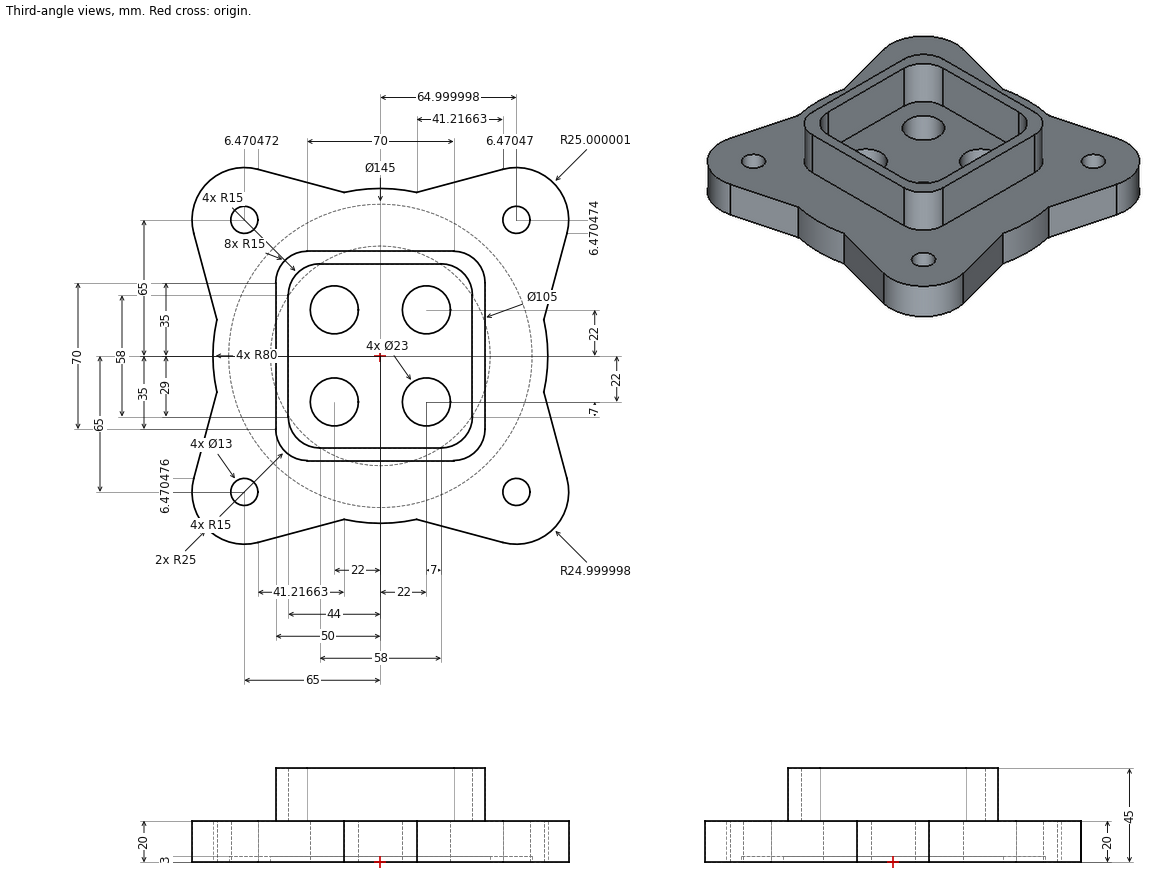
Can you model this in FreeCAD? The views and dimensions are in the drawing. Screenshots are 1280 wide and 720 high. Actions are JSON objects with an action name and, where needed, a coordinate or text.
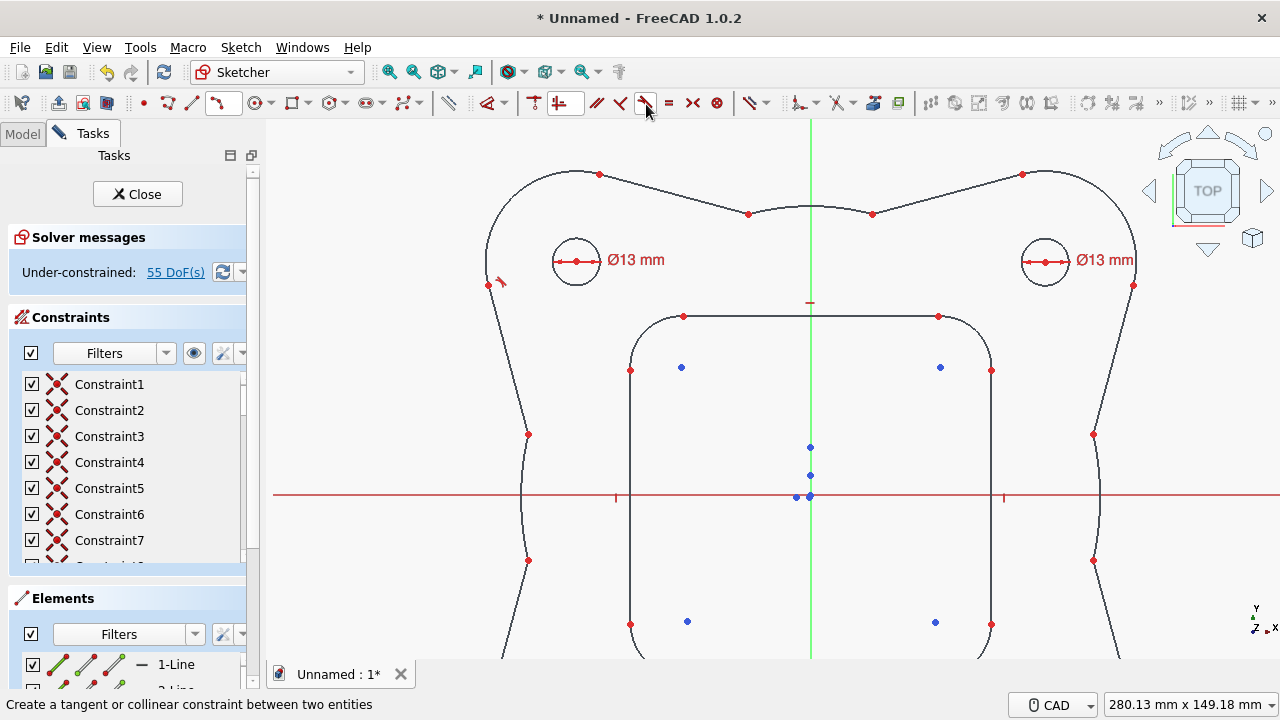
{"action": "left_click", "coordinate": [516, 605]}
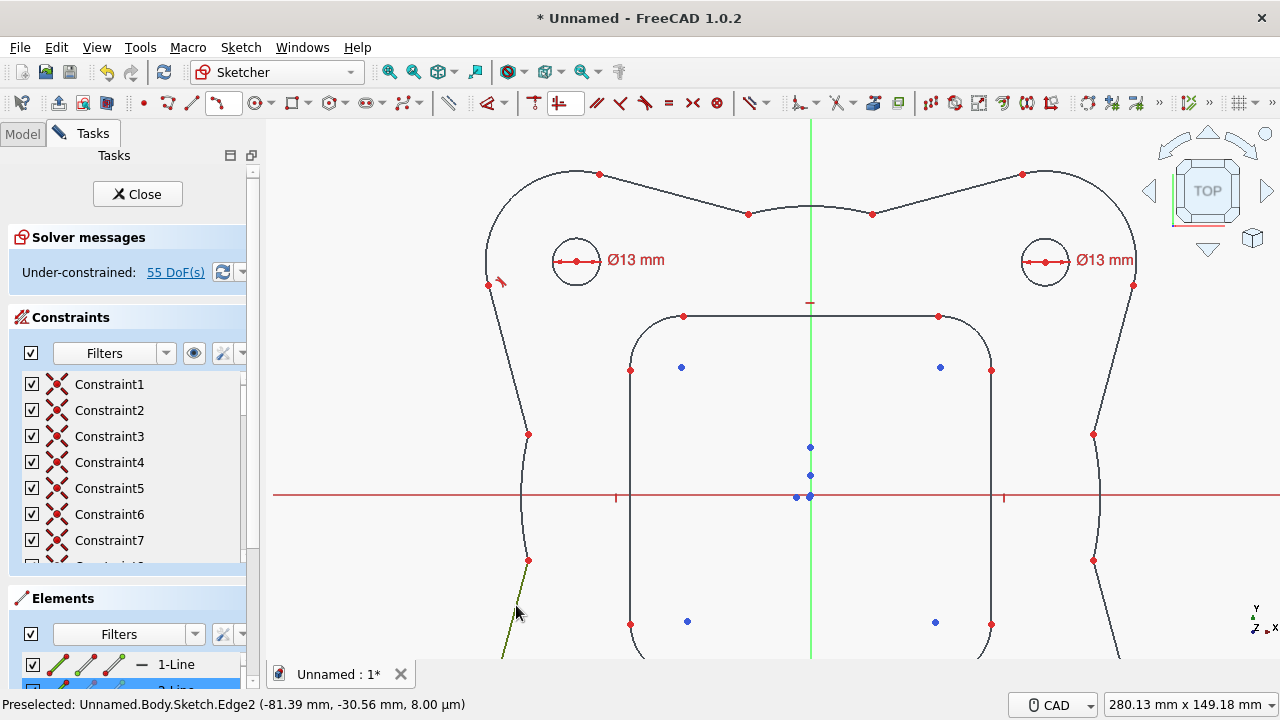
{"action": "scroll", "coordinate": [575, 260], "scroll_direction": "down", "scroll_amount": 3}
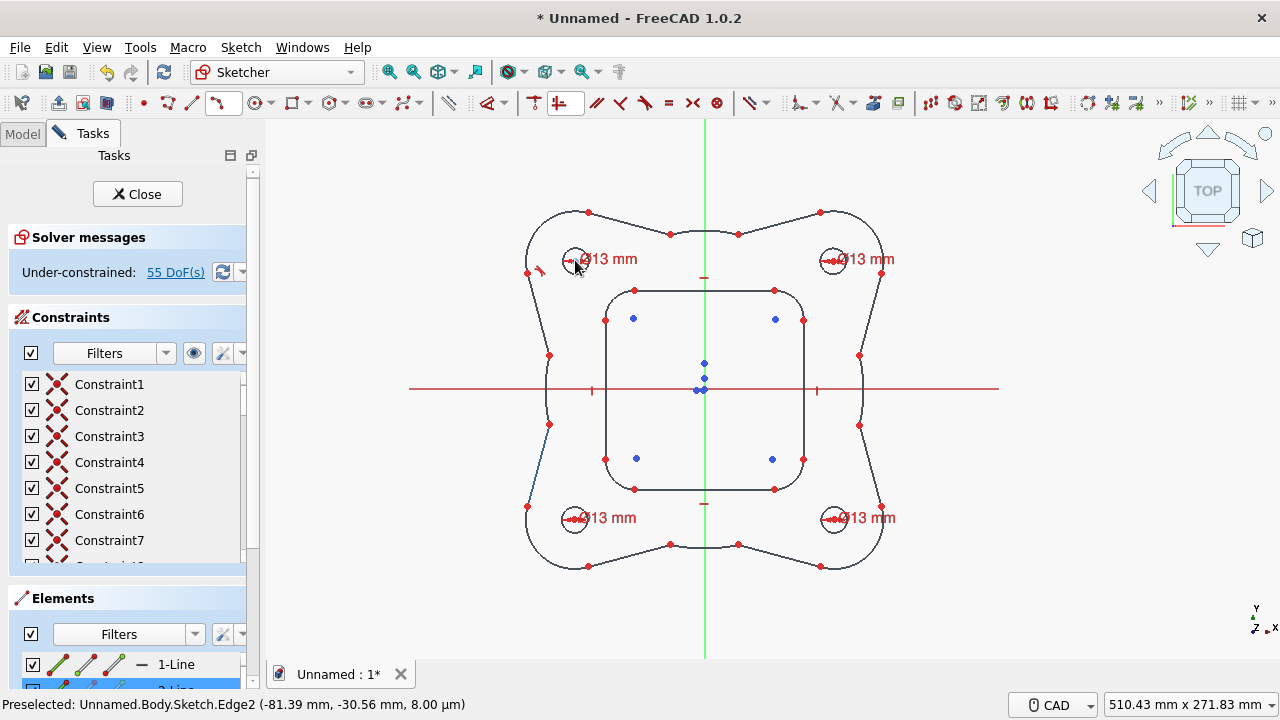
{"action": "left_click", "coordinate": [529, 538]}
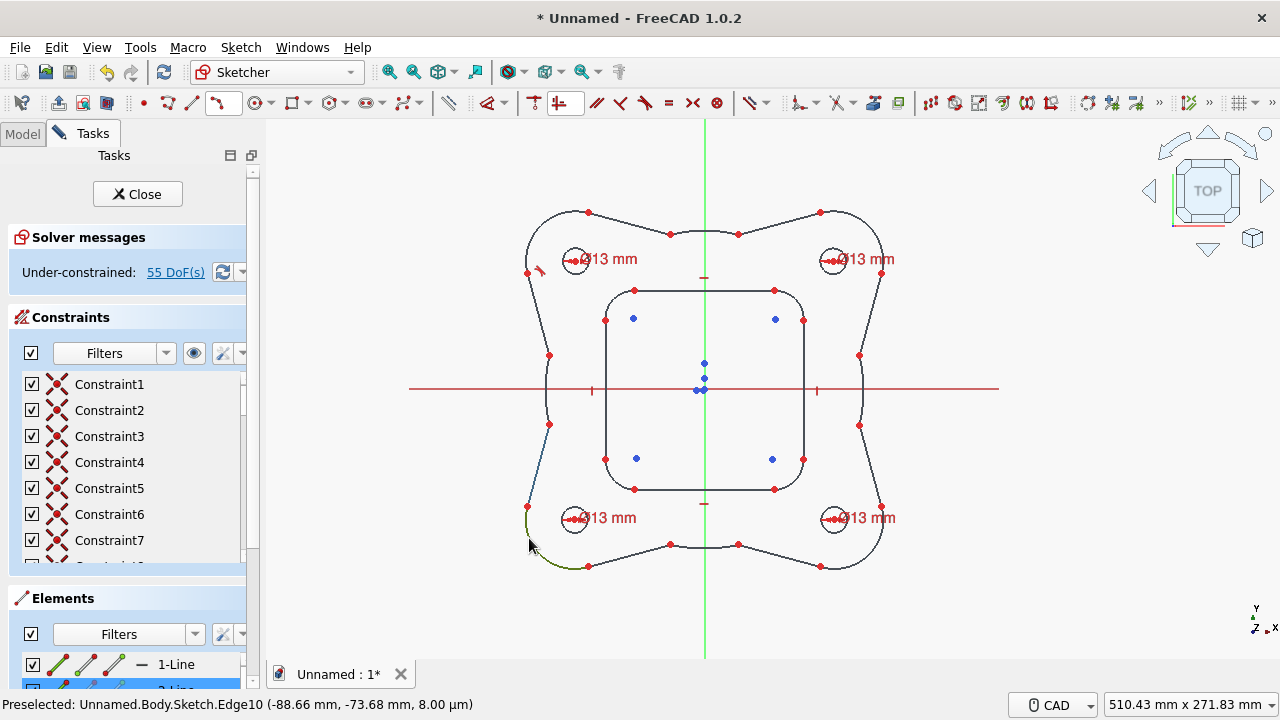
{"action": "left_click", "coordinate": [646, 104]}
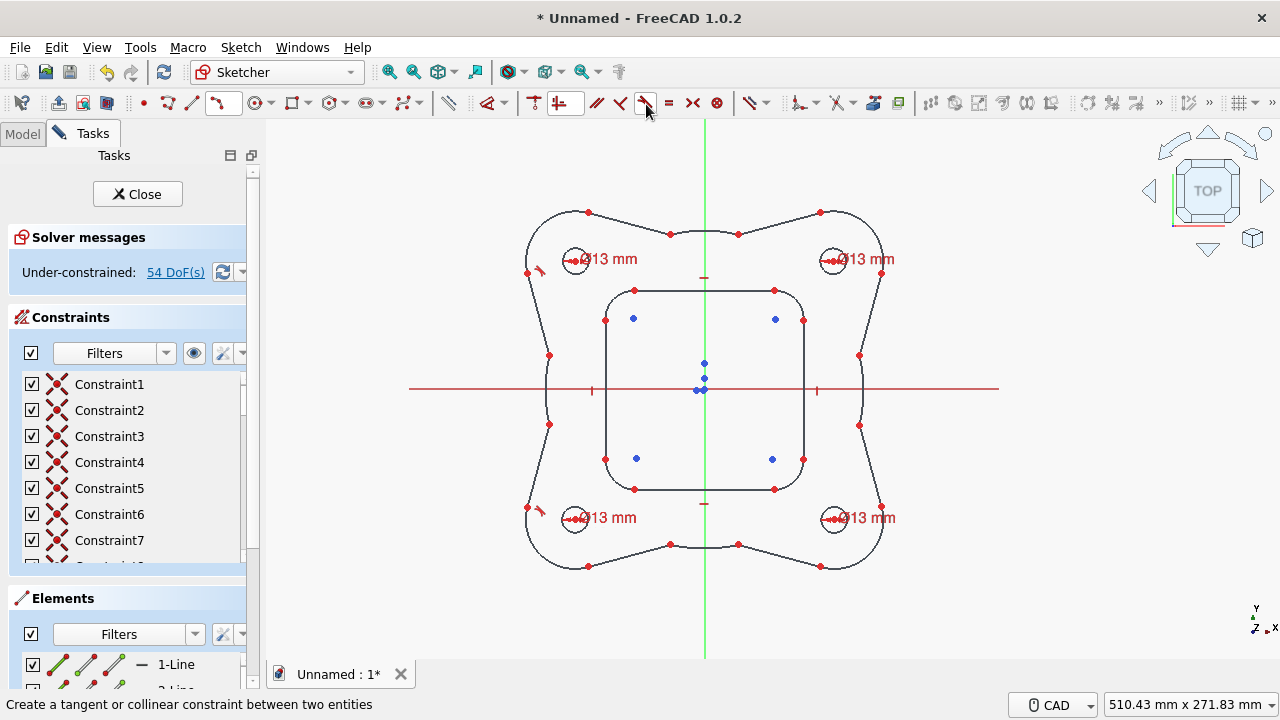
{"action": "left_click", "coordinate": [613, 560]}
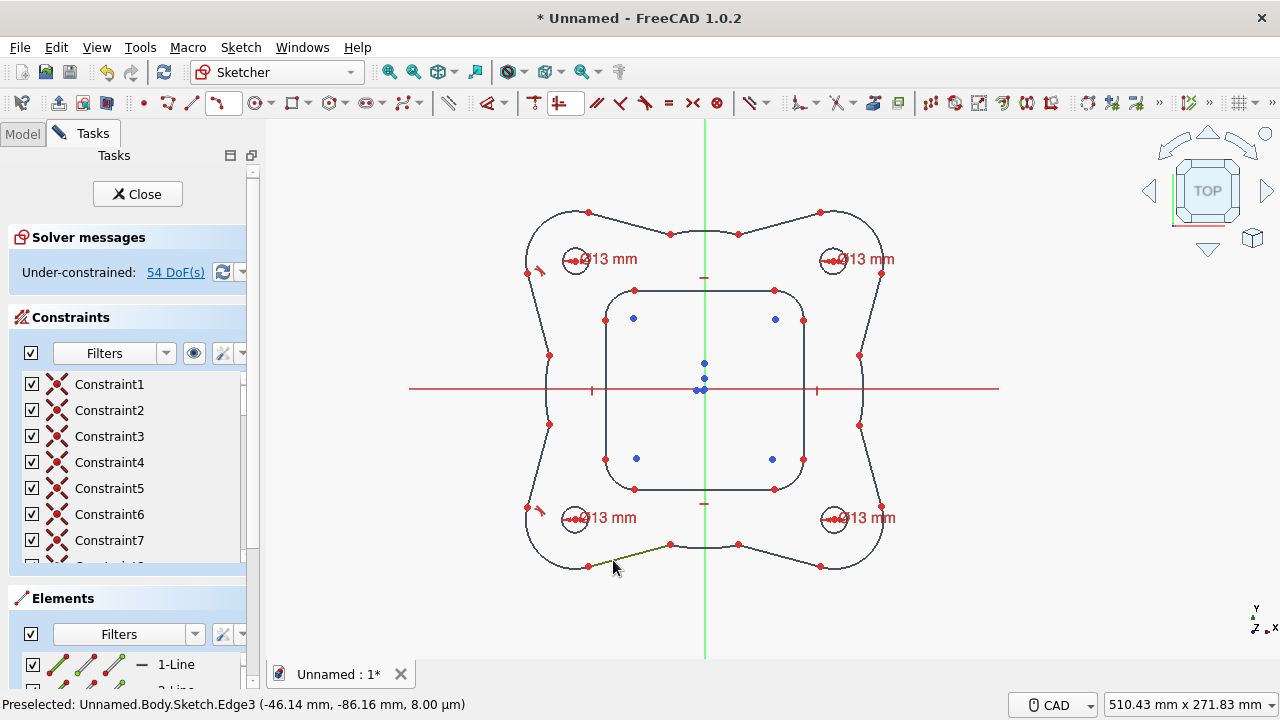
{"action": "left_click", "coordinate": [529, 538]}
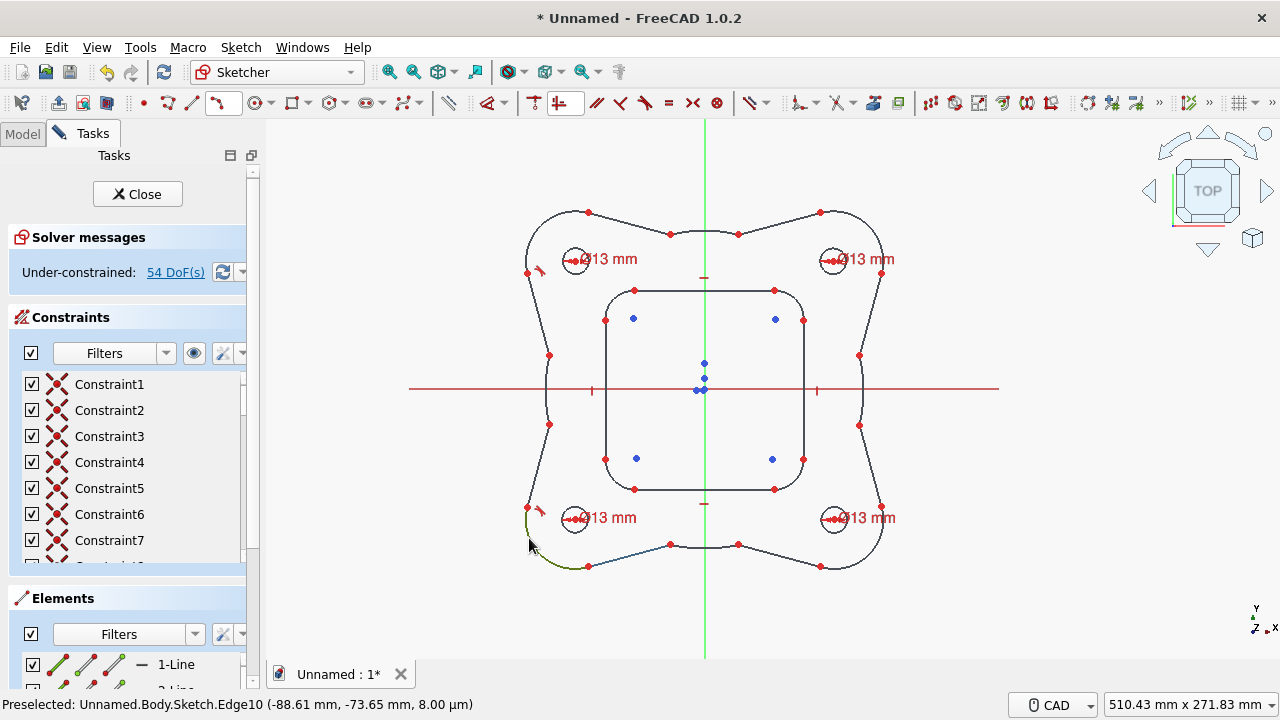
{"action": "key", "text": "t"}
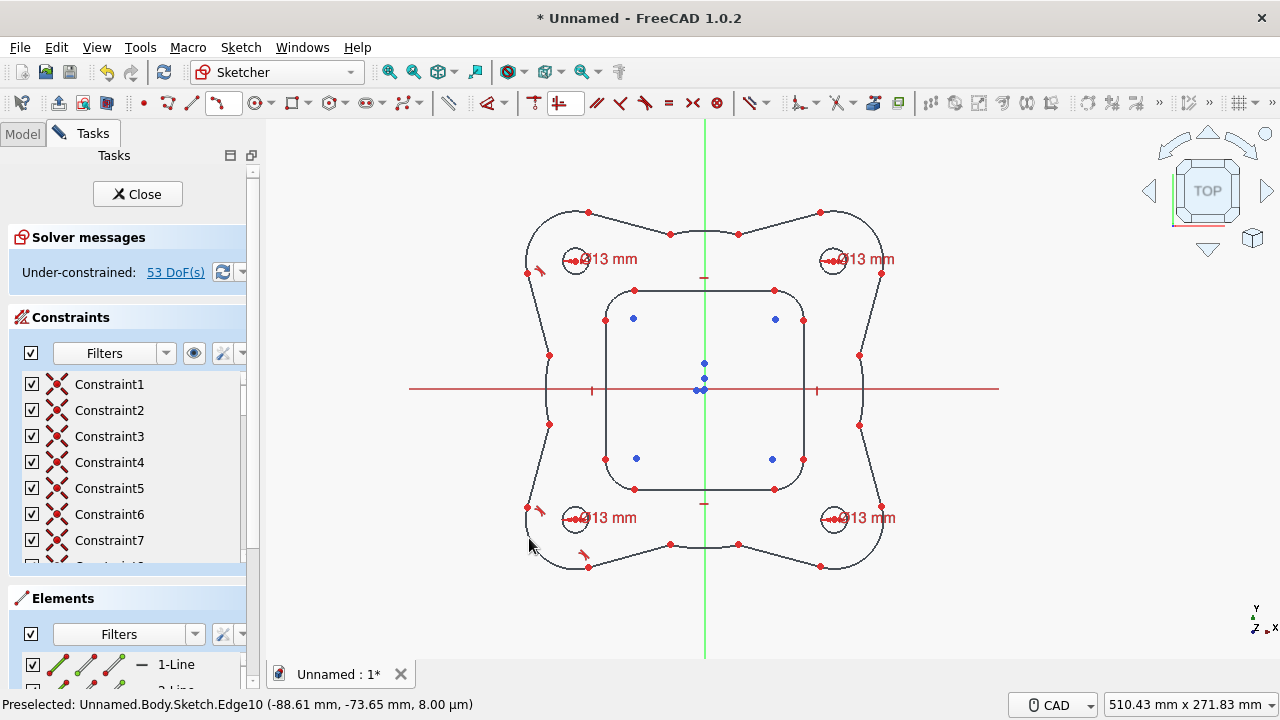
{"action": "left_click", "coordinate": [763, 552]}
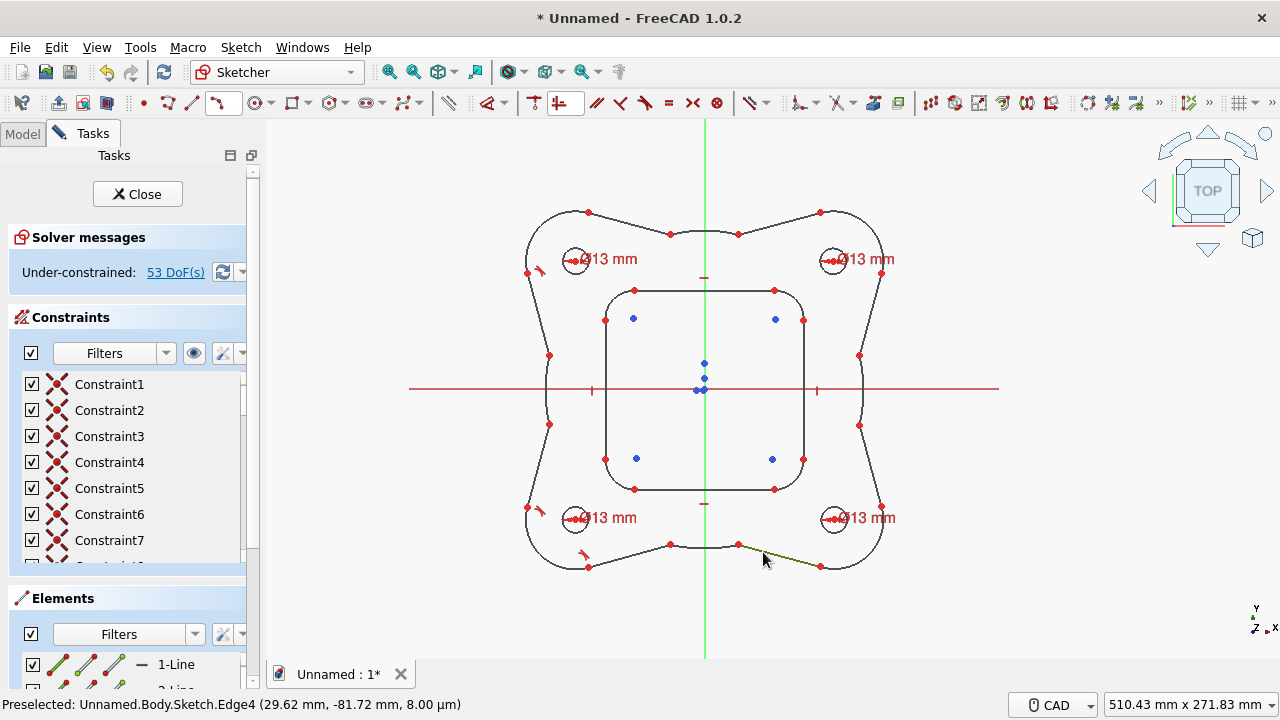
{"action": "left_click", "coordinate": [851, 566]}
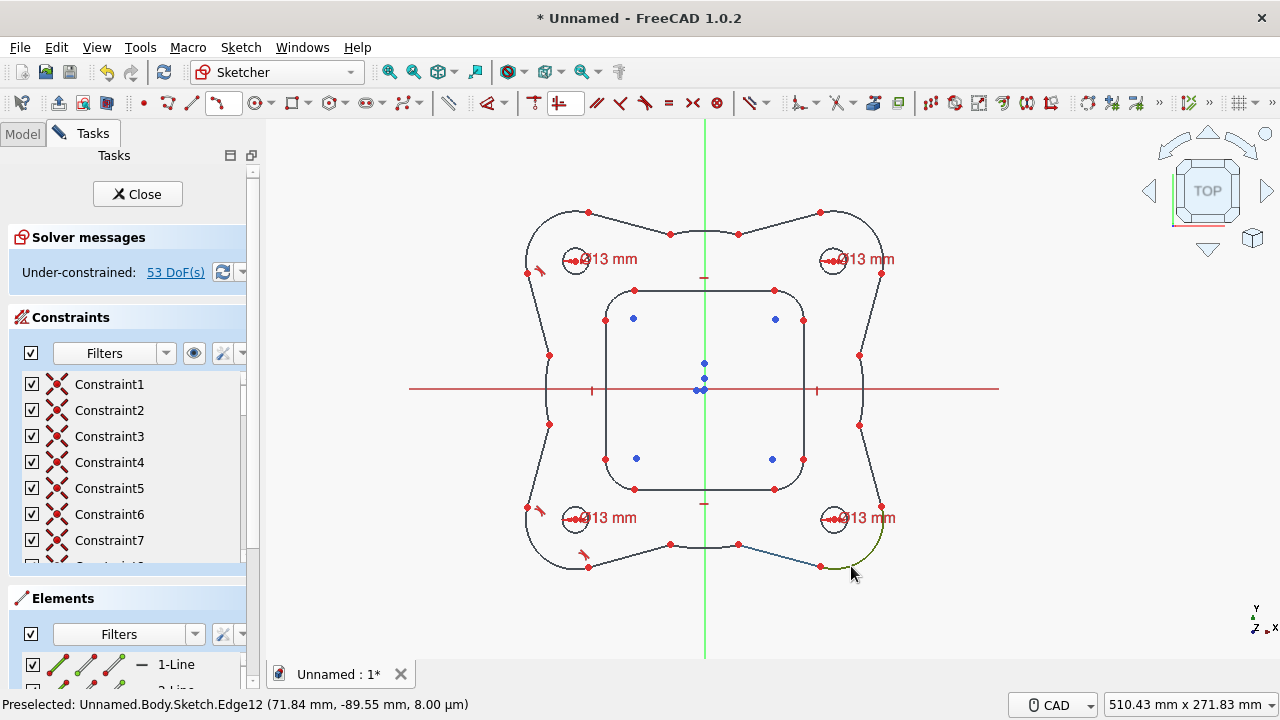
{"action": "left_click", "coordinate": [646, 104]}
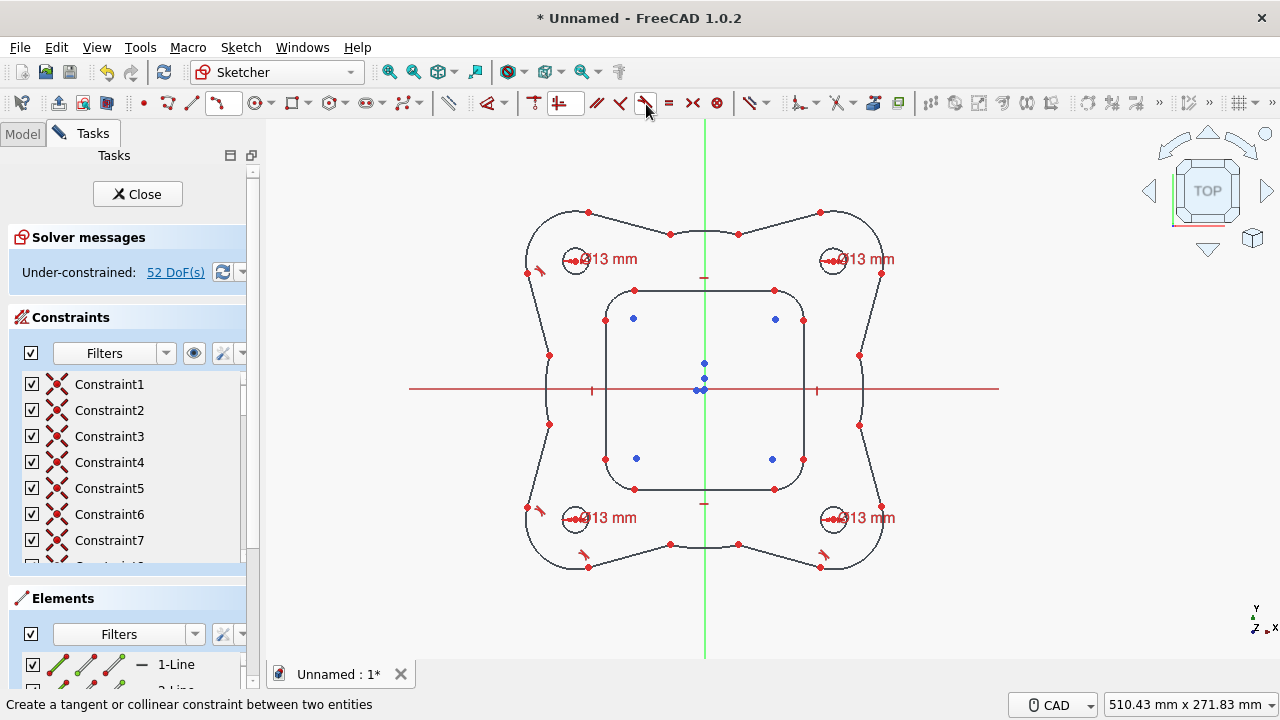
{"action": "left_click", "coordinate": [875, 482]}